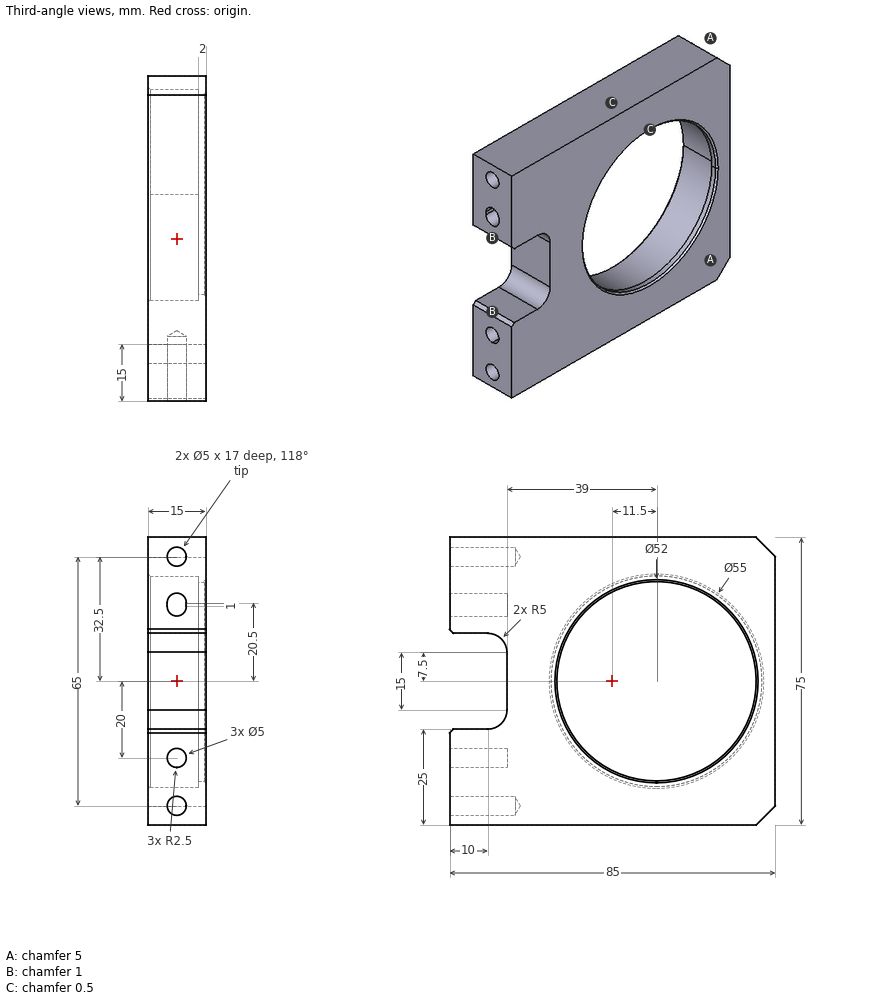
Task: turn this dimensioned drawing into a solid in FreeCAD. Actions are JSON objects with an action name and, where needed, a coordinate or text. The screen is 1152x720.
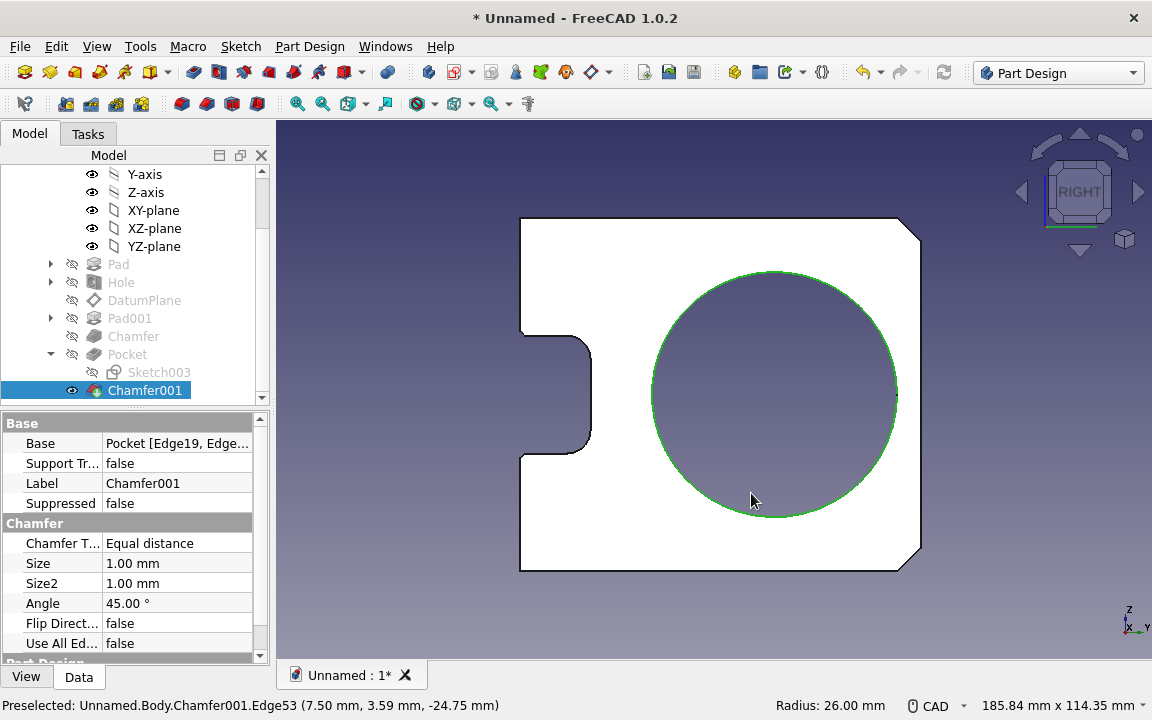
{"action": "key", "text": "5"}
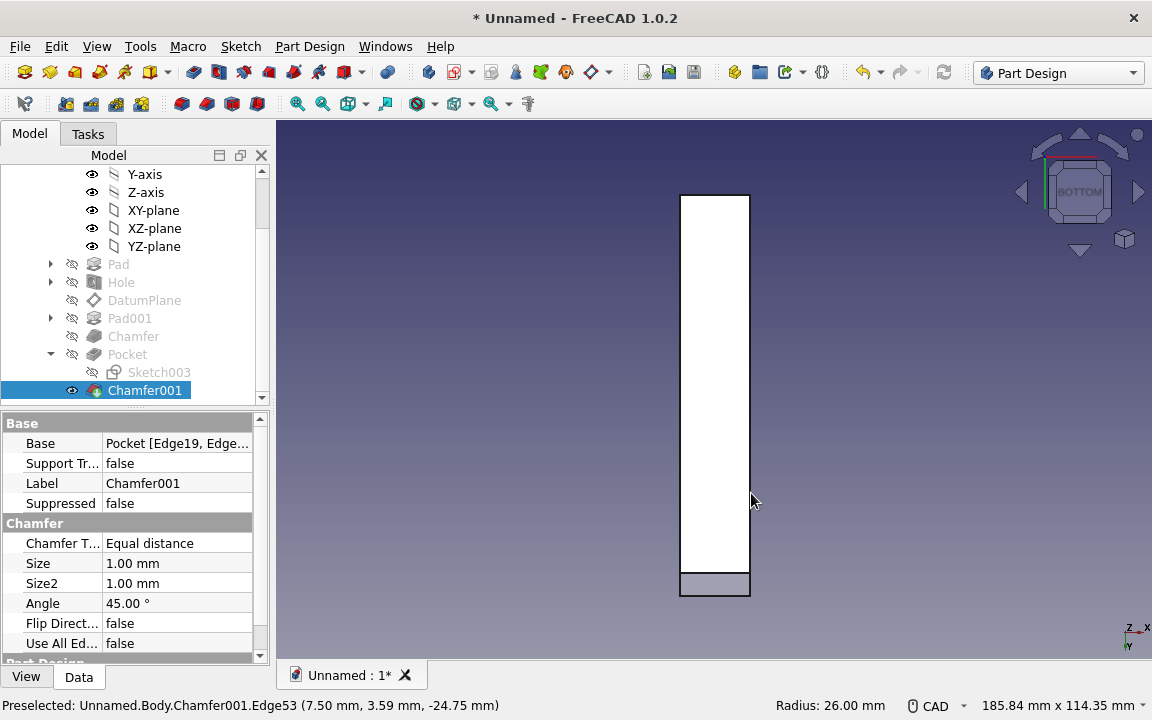
{"action": "key", "text": "4"}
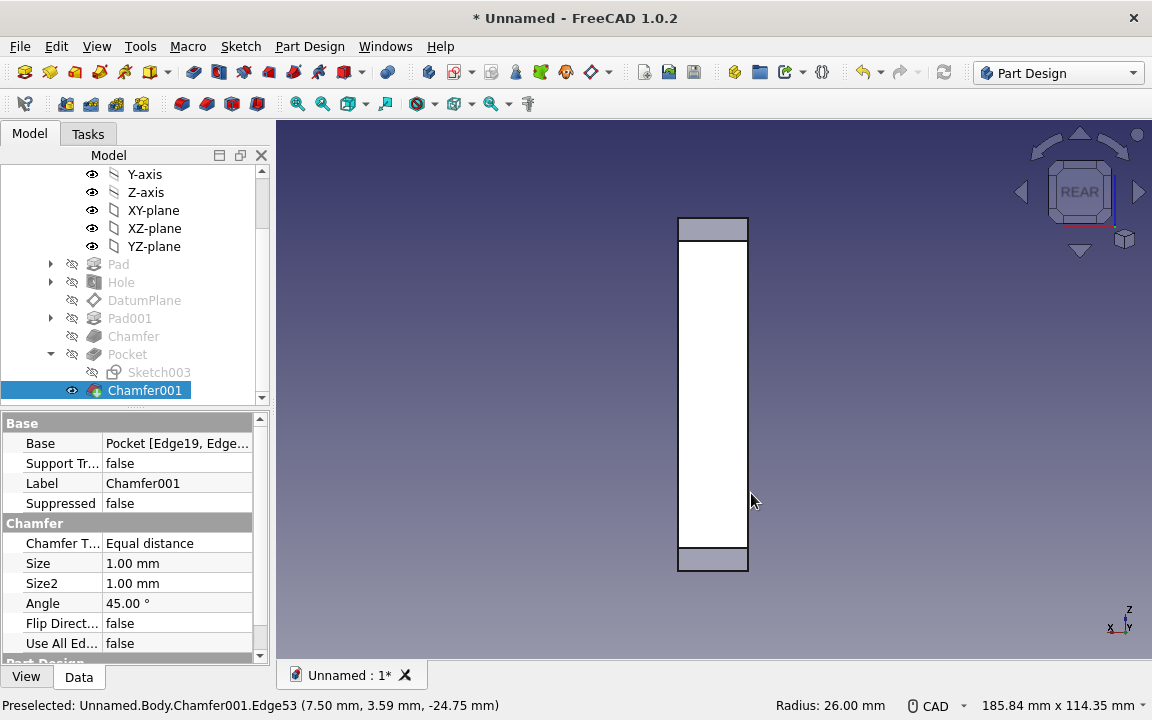
{"action": "key", "text": "6"}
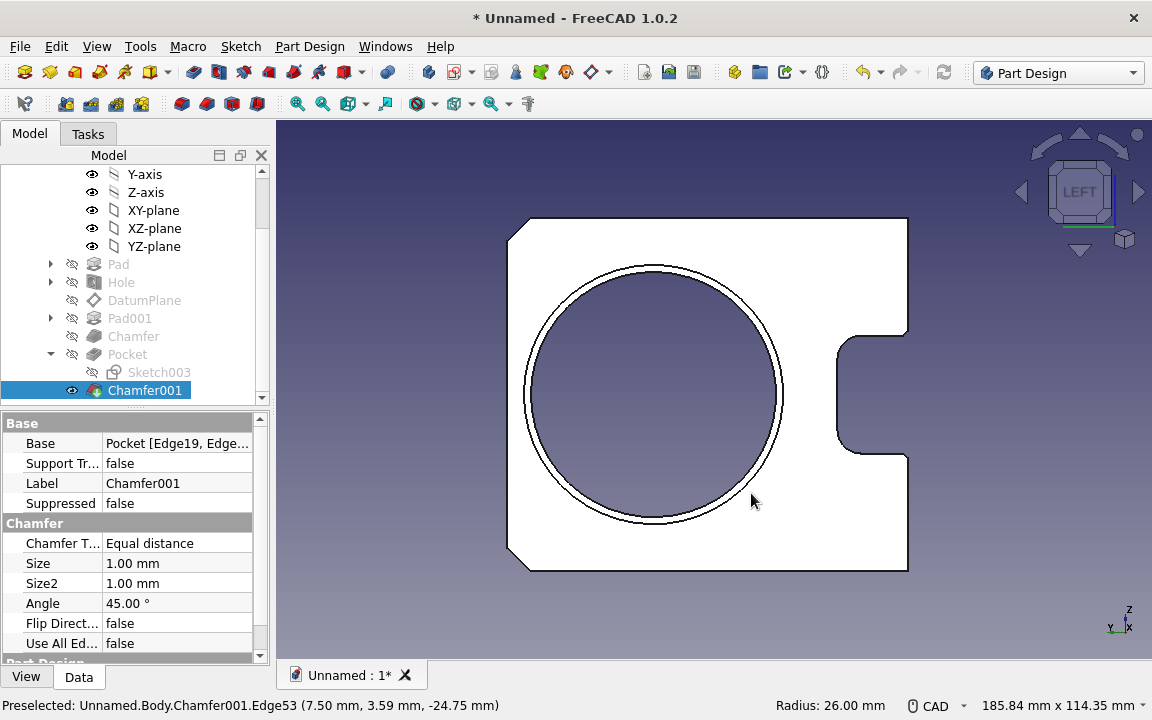
{"action": "left_click", "coordinate": [783, 394], "text": "ctrl"}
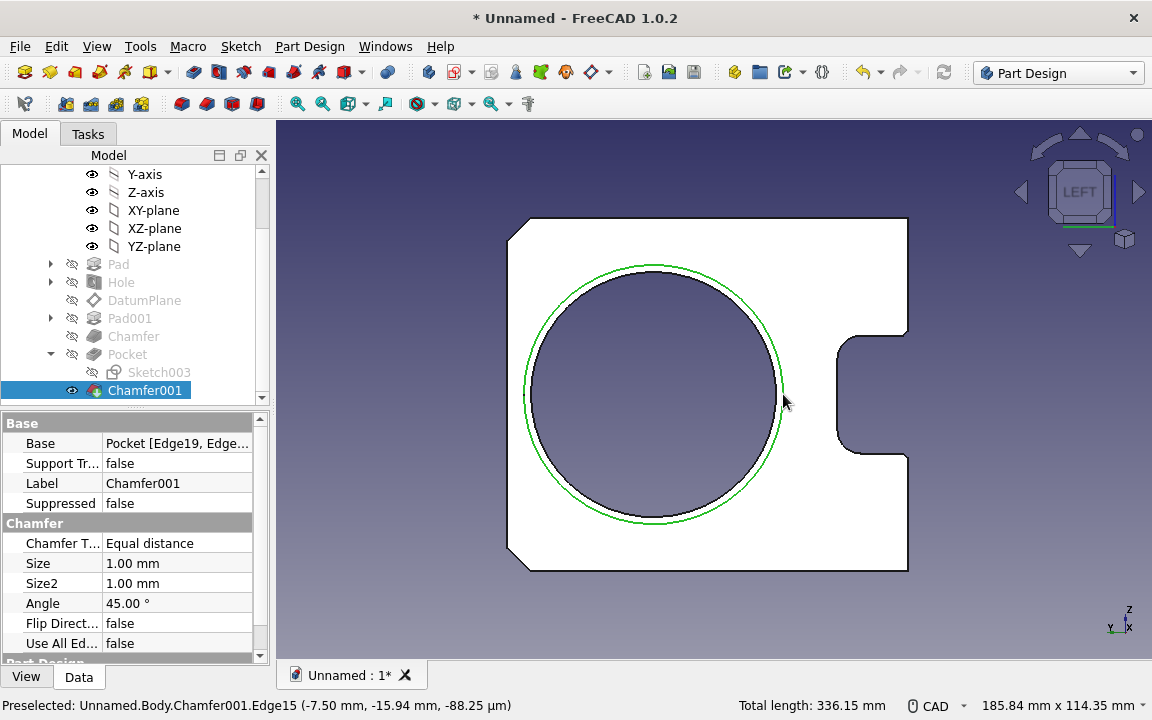
{"action": "left_click", "coordinate": [207, 104]}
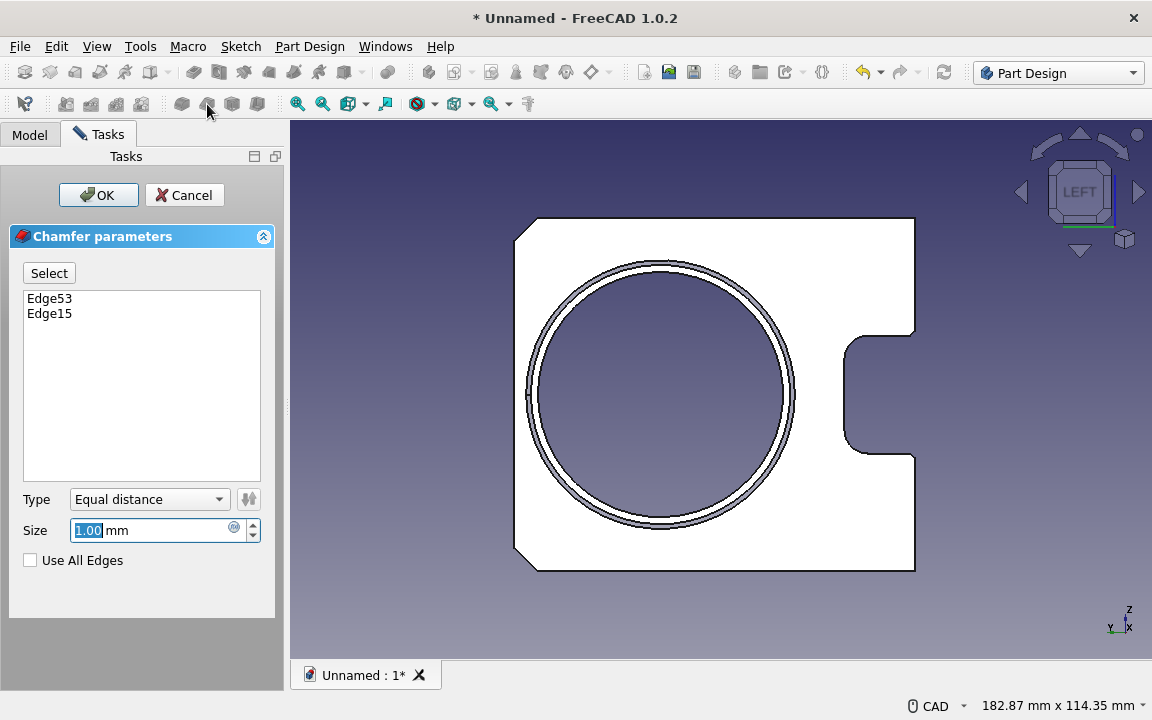
{"action": "type", "text": "0.5"}
{"action": "key", "text": "Tab"}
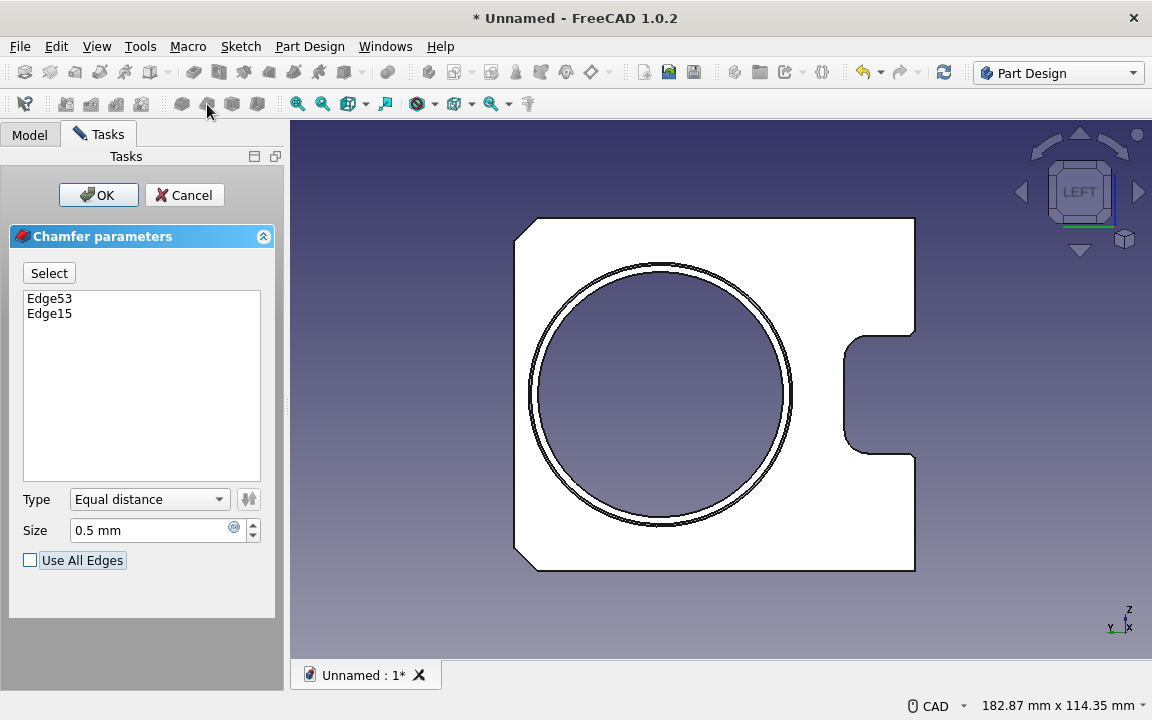
{"action": "left_click", "coordinate": [99, 195]}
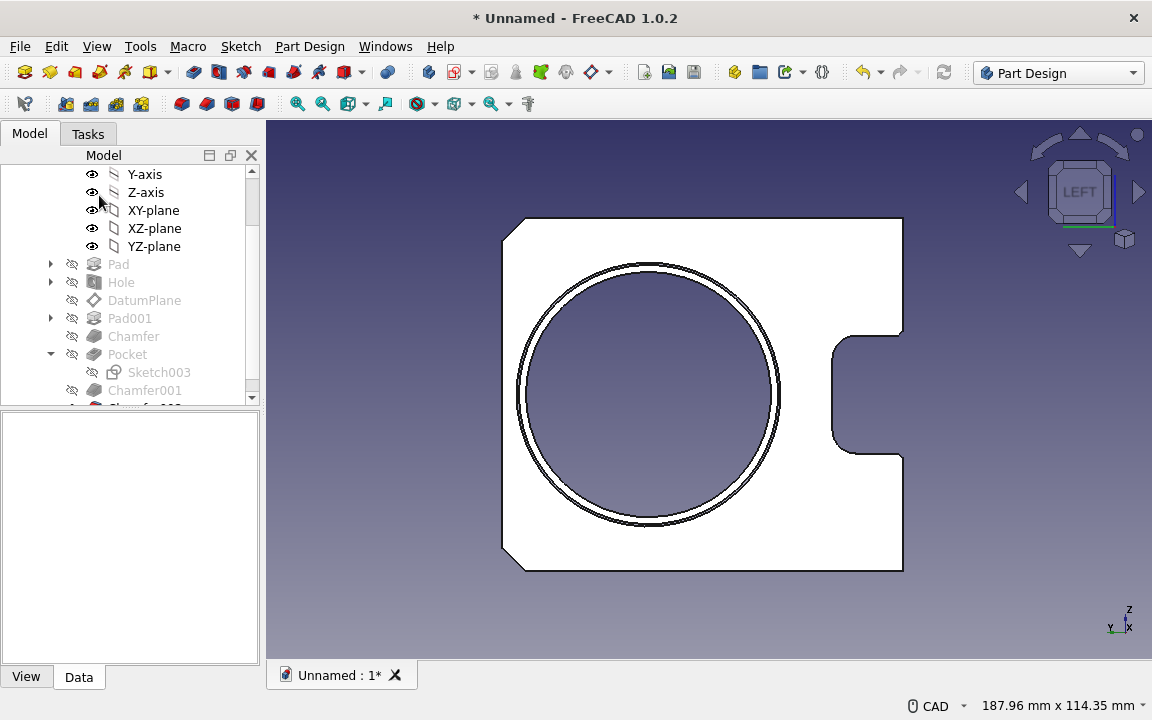
{"action": "key", "text": "0"}